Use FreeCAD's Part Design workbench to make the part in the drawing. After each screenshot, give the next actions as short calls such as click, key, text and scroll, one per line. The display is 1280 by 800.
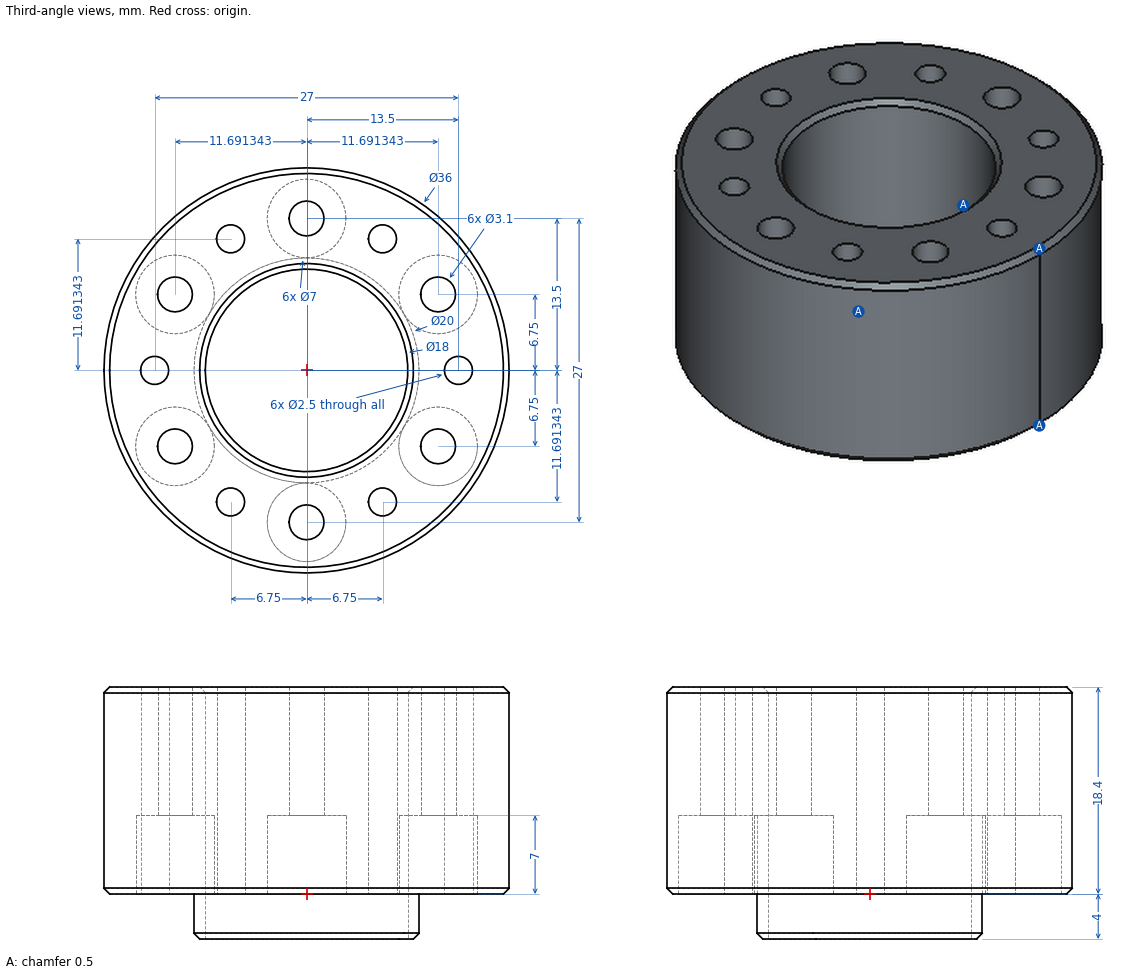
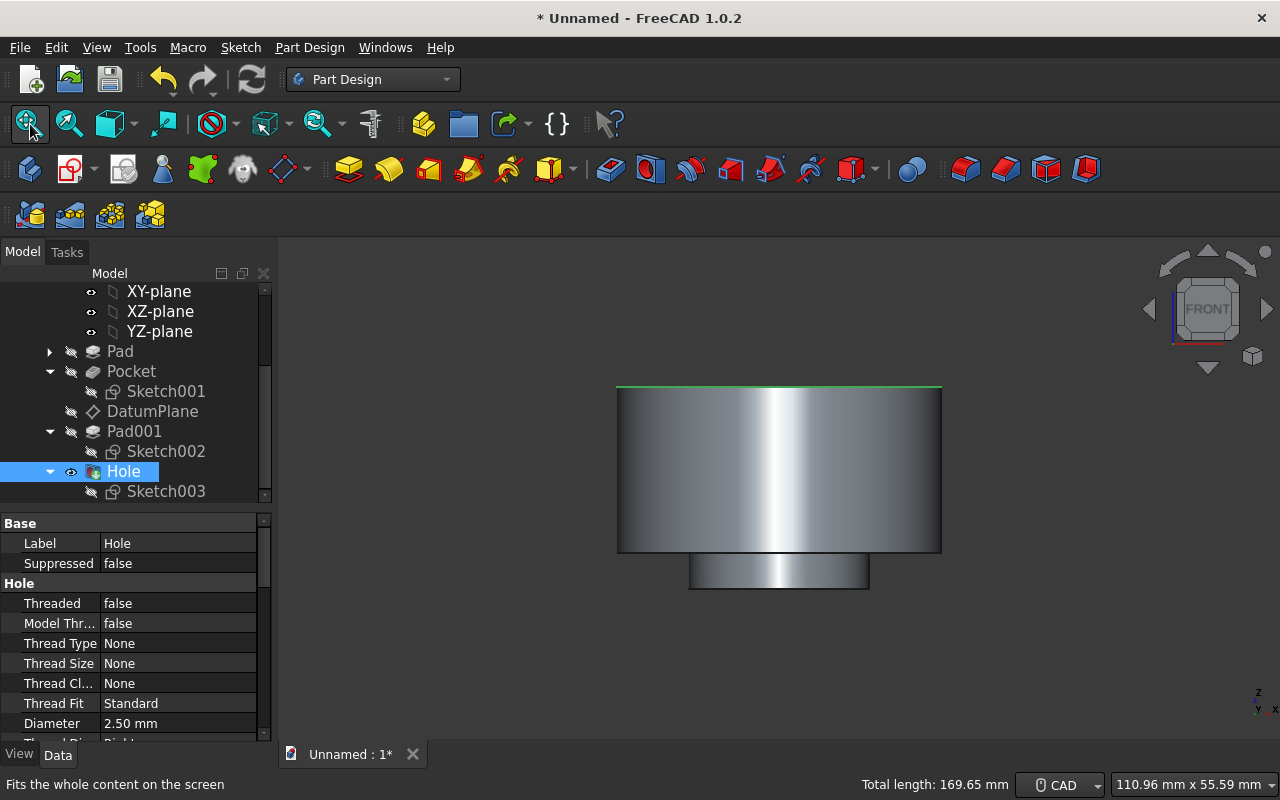
click(647, 552, ctrl)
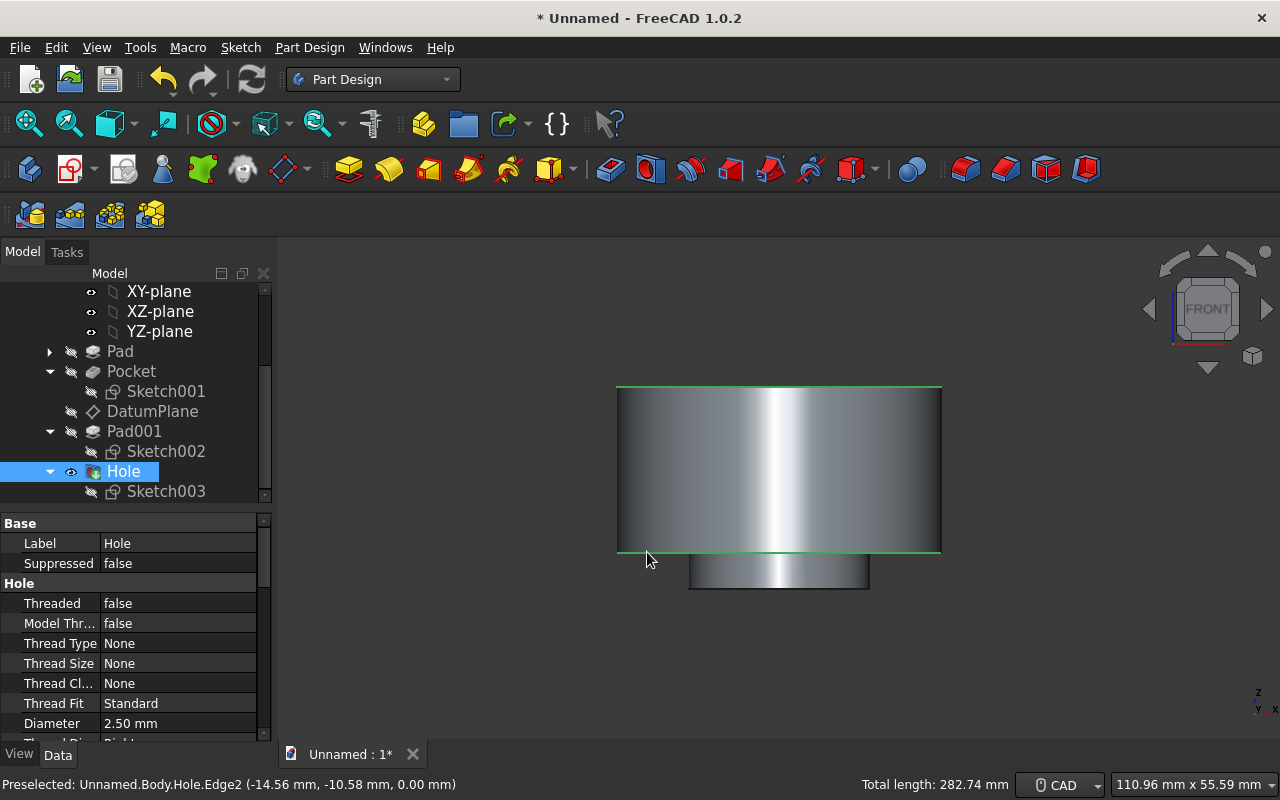
click(845, 588, ctrl)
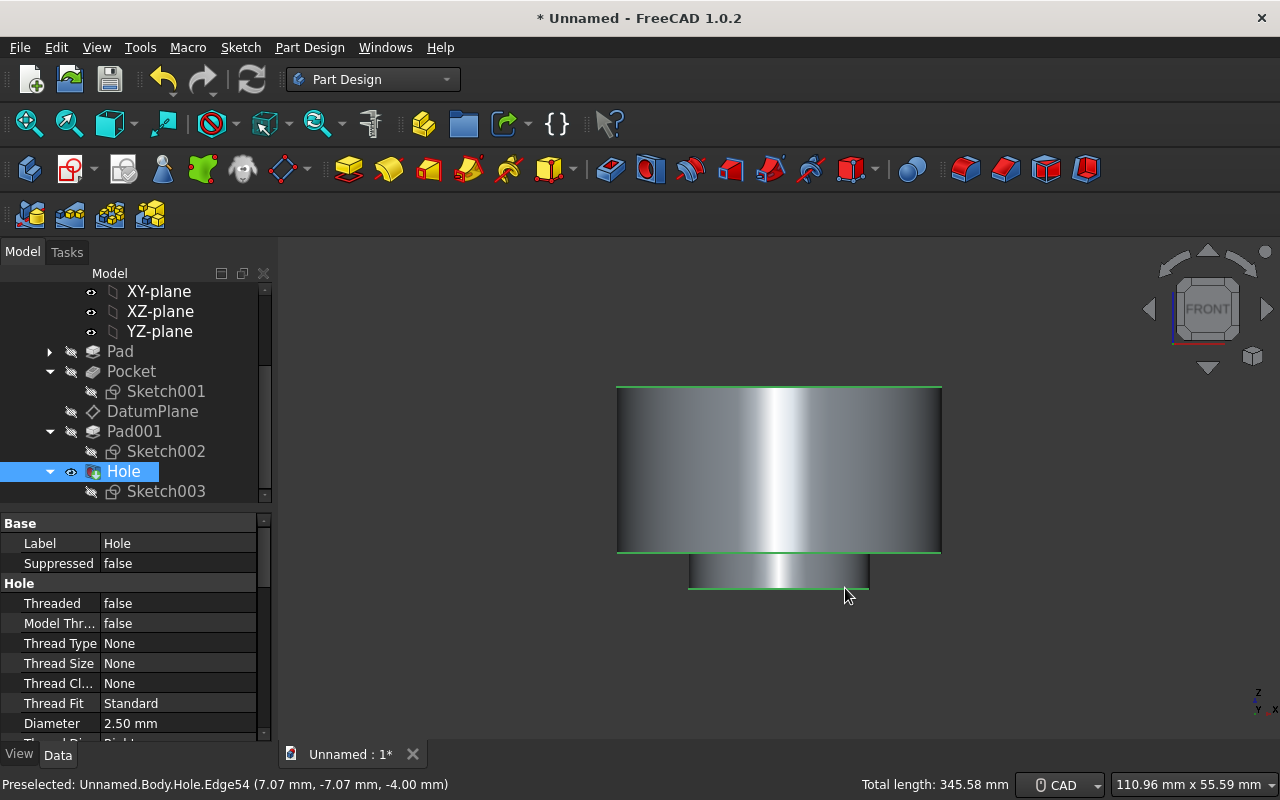
click(1006, 170)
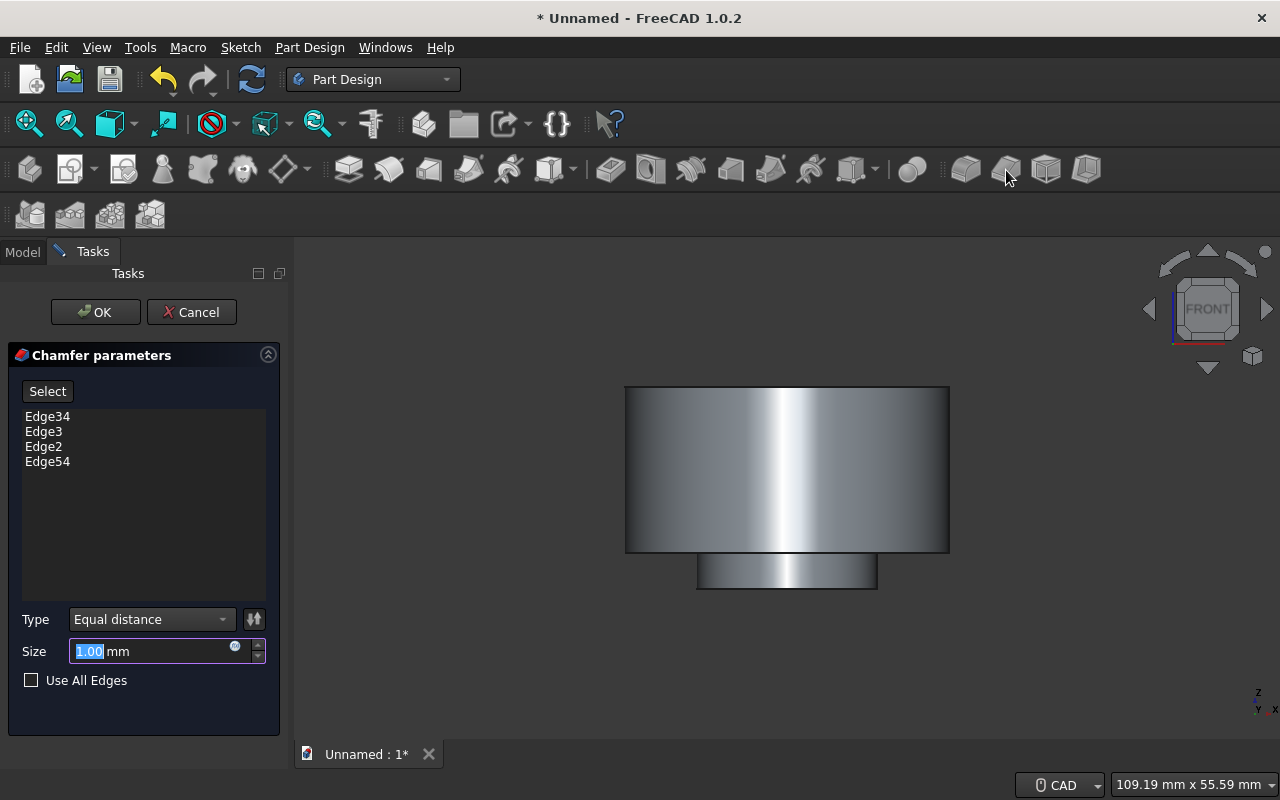
text(0.5)
key(Tab)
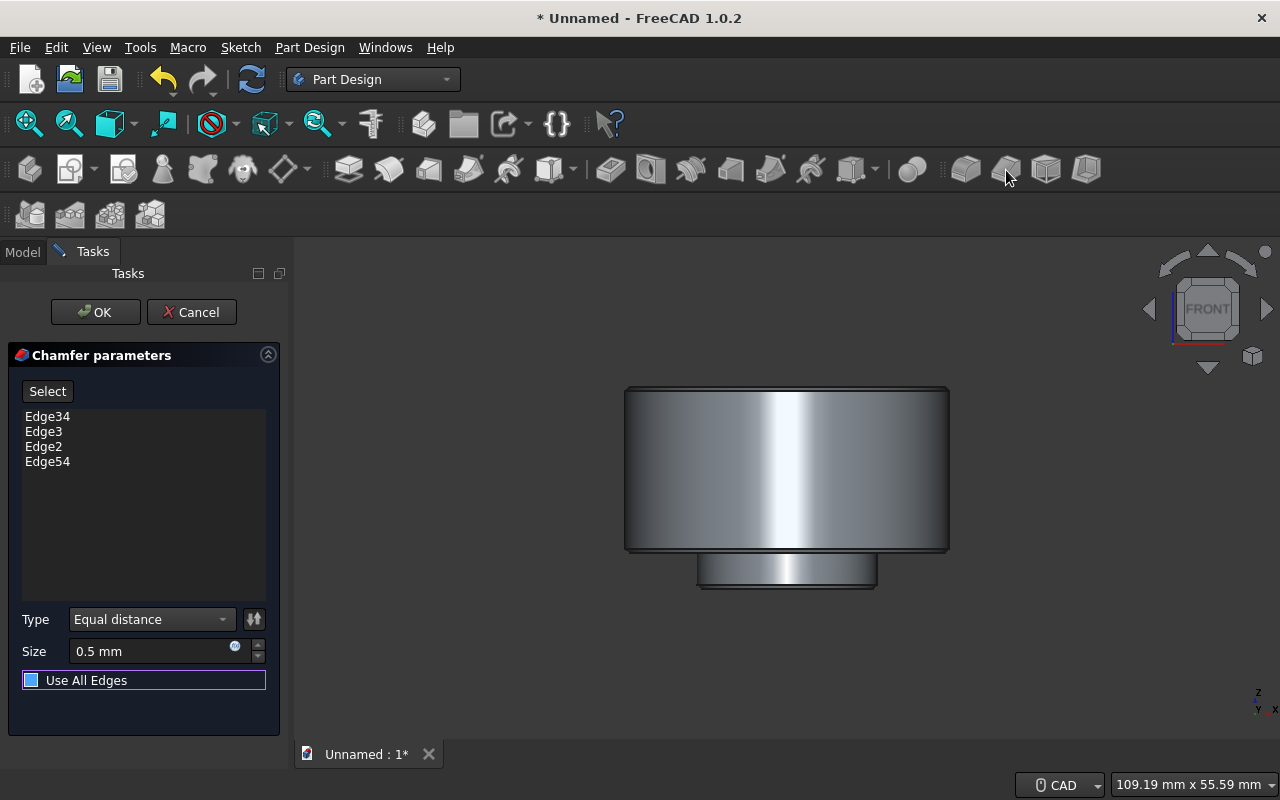
click(96, 312)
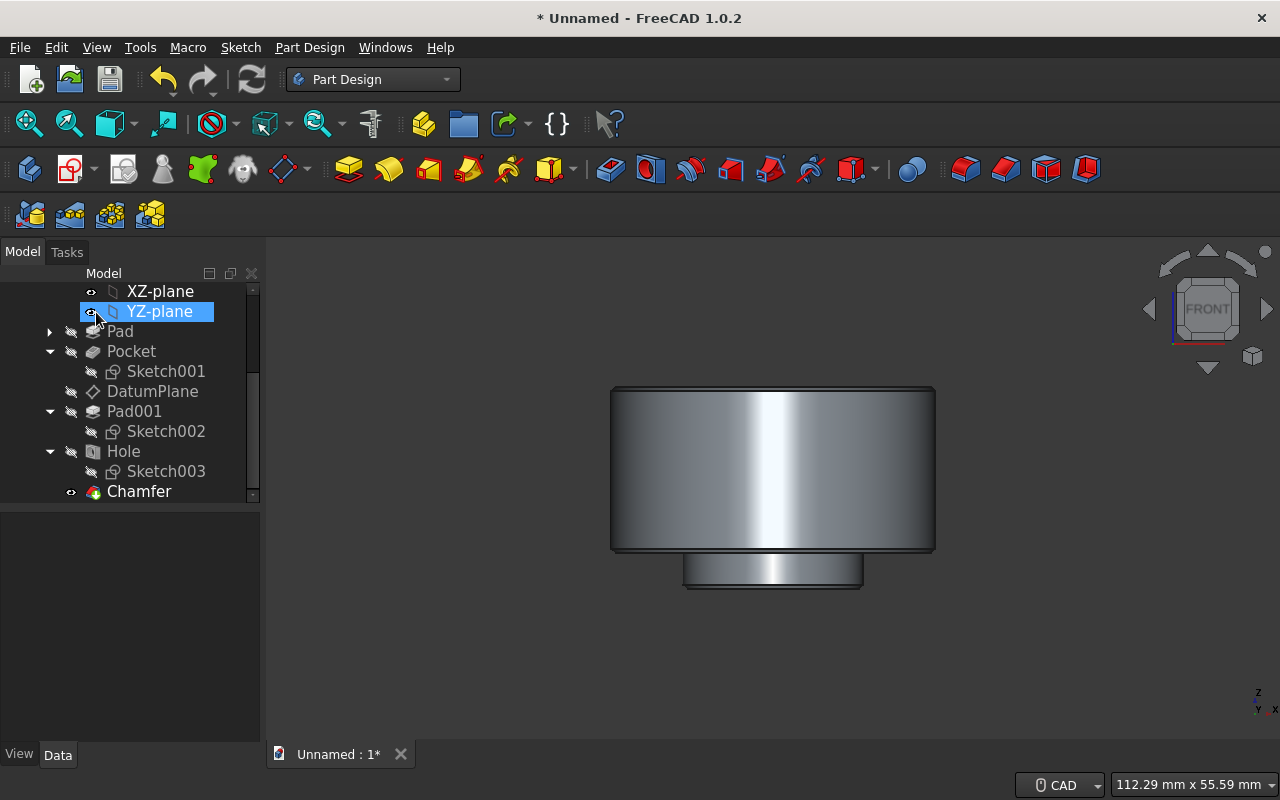
key(0)